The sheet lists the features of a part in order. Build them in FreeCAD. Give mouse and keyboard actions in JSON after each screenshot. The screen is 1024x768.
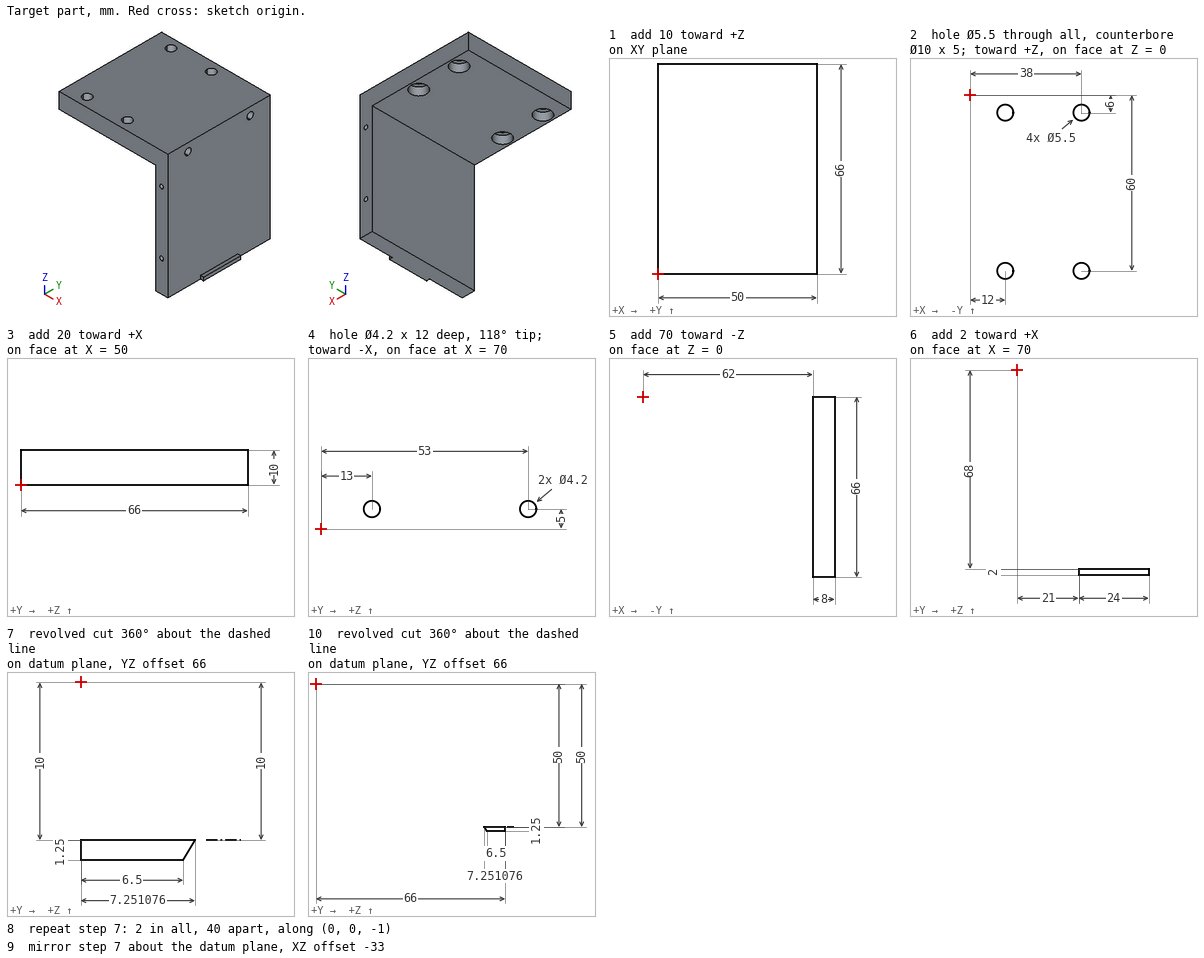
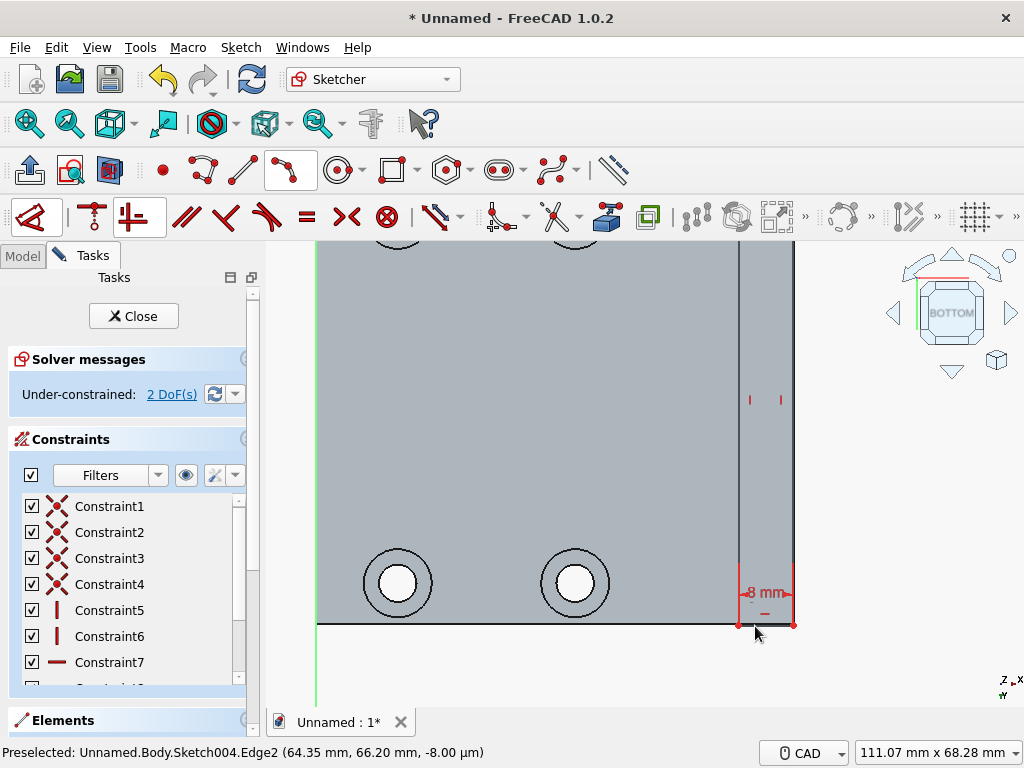
{"action": "left_click", "coordinate": [739, 309]}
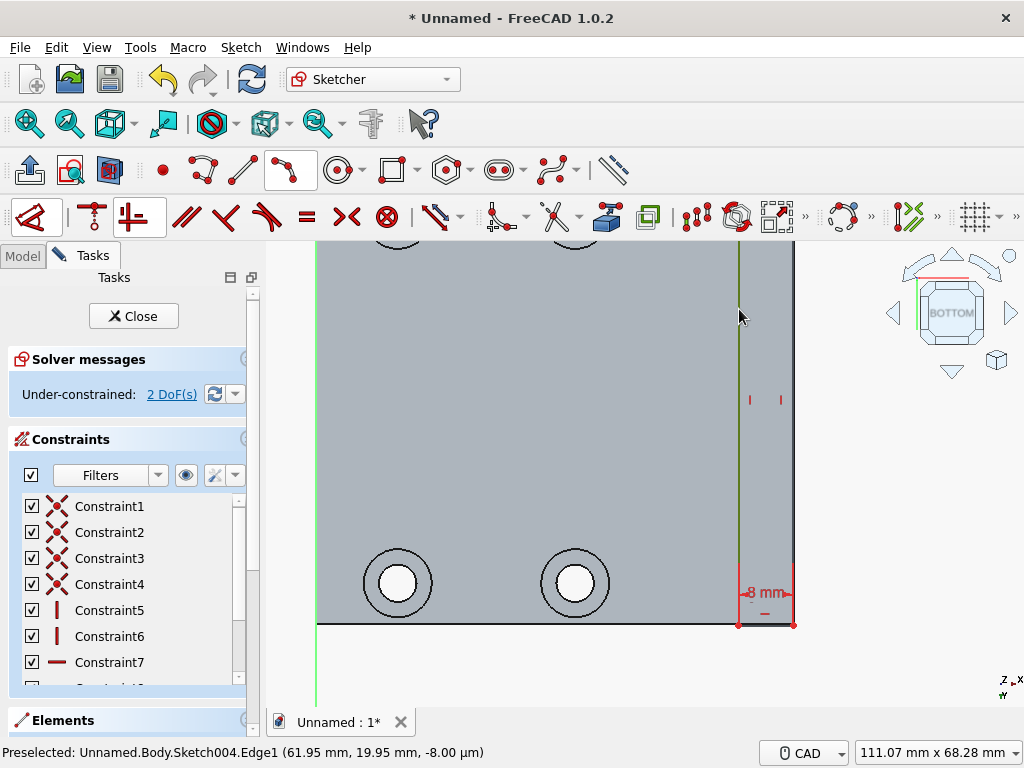
{"action": "key", "text": "i"}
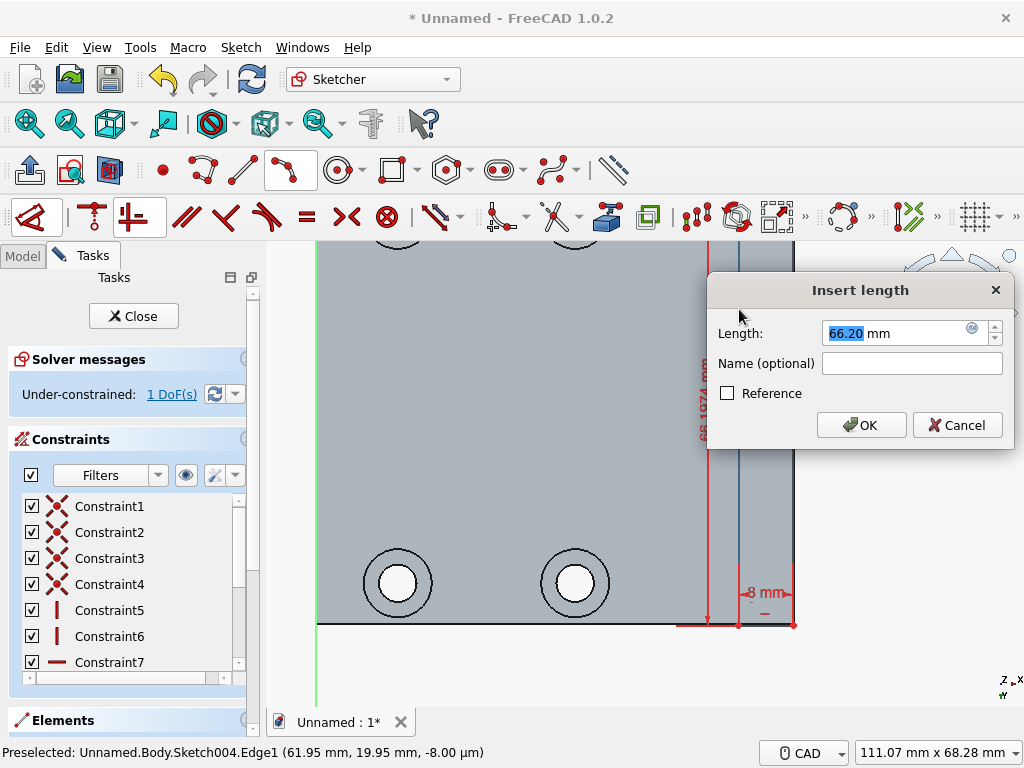
{"action": "type", "text": "66"}
{"action": "key", "text": "Return"}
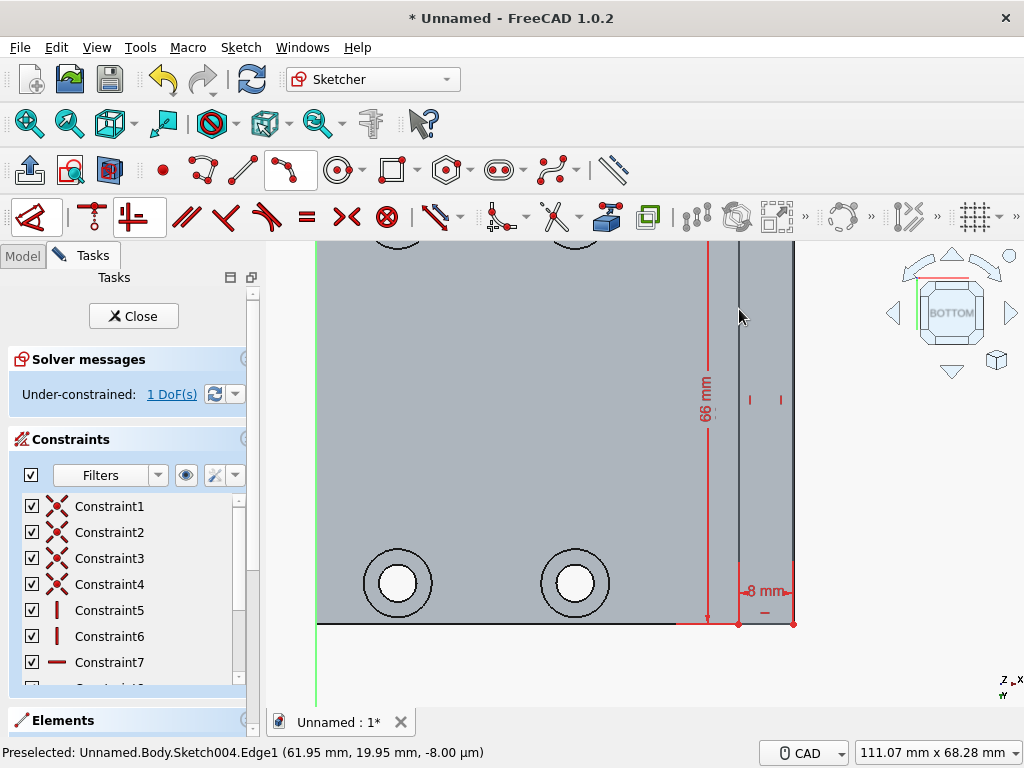
{"action": "scroll", "coordinate": [621, 626], "scroll_direction": "down", "scroll_amount": 2}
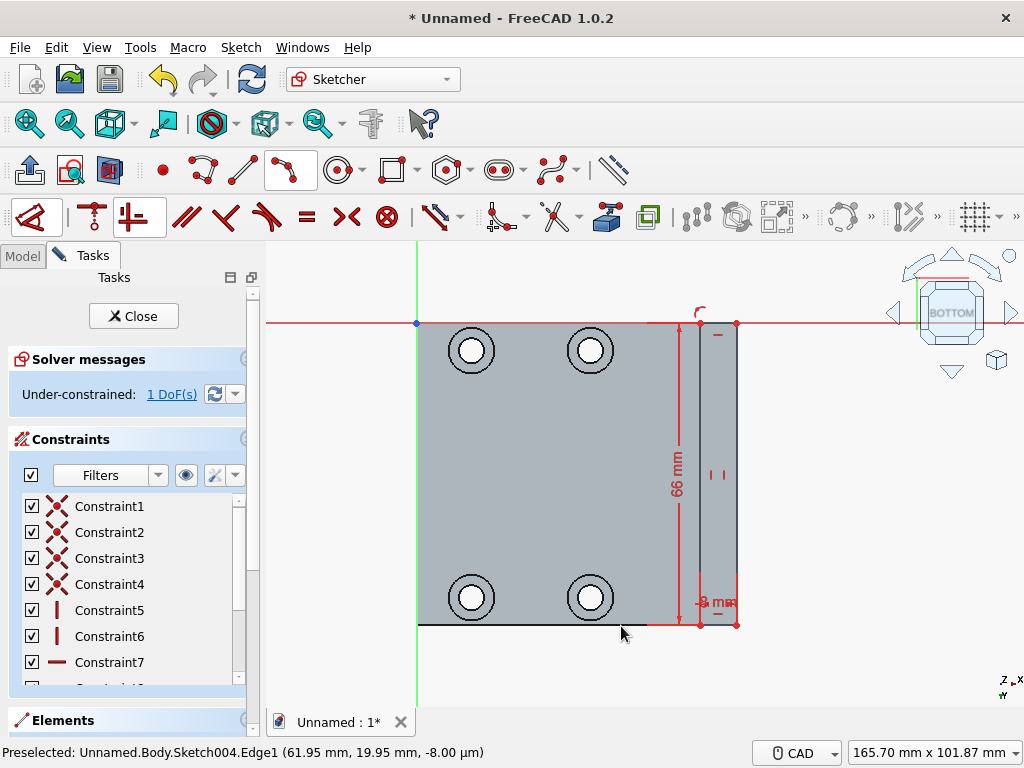
{"action": "left_click", "coordinate": [700, 323]}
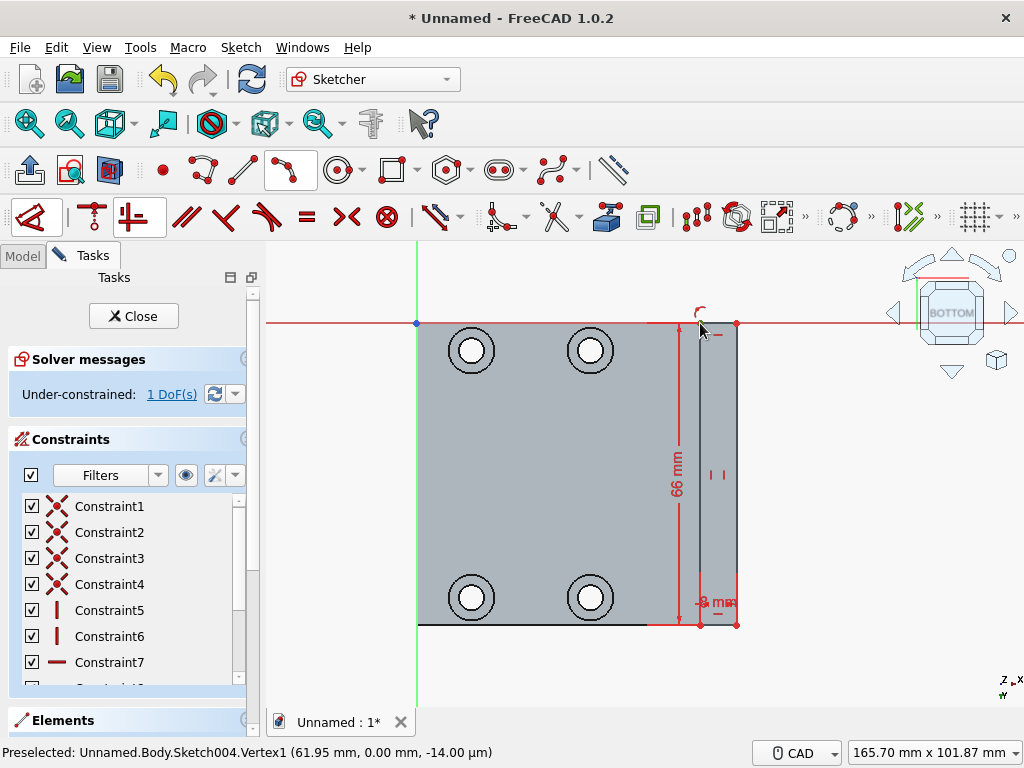
{"action": "key", "text": "l"}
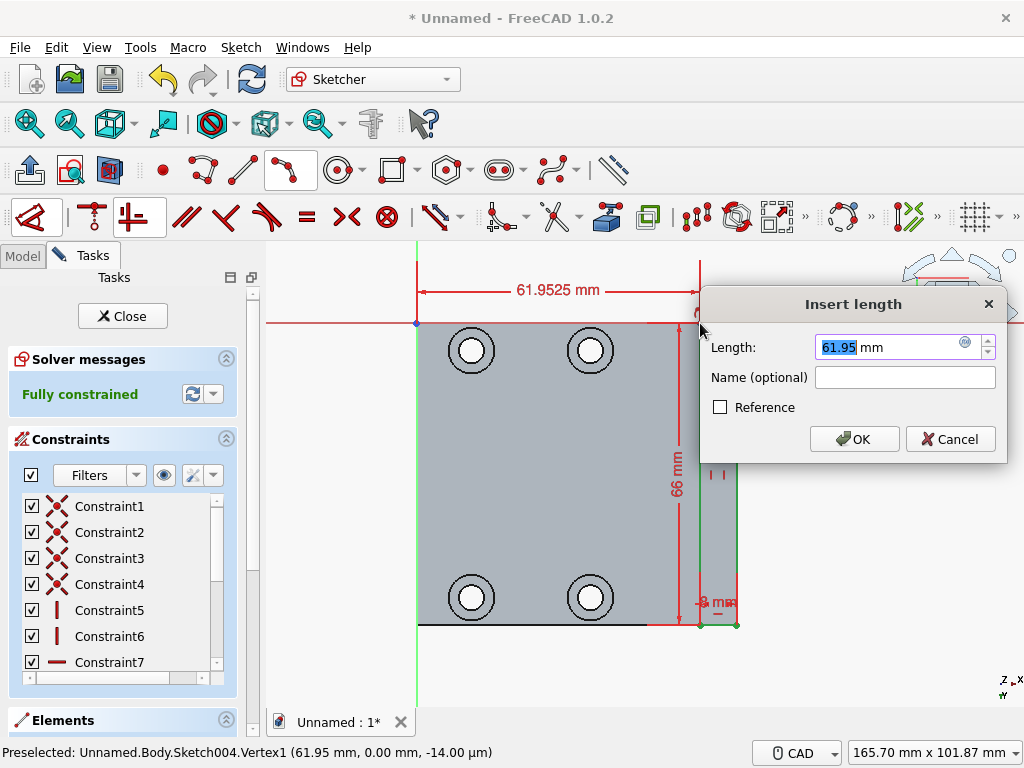
{"action": "type", "text": "62"}
{"action": "key", "text": "Return"}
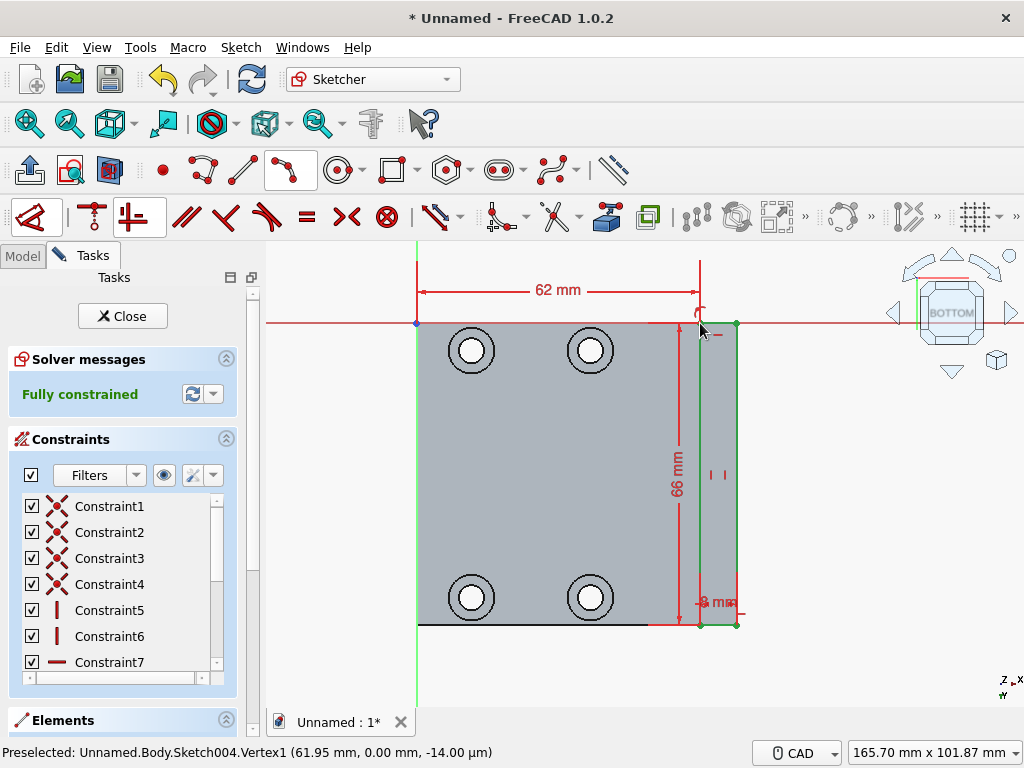
{"action": "left_click", "coordinate": [123, 316]}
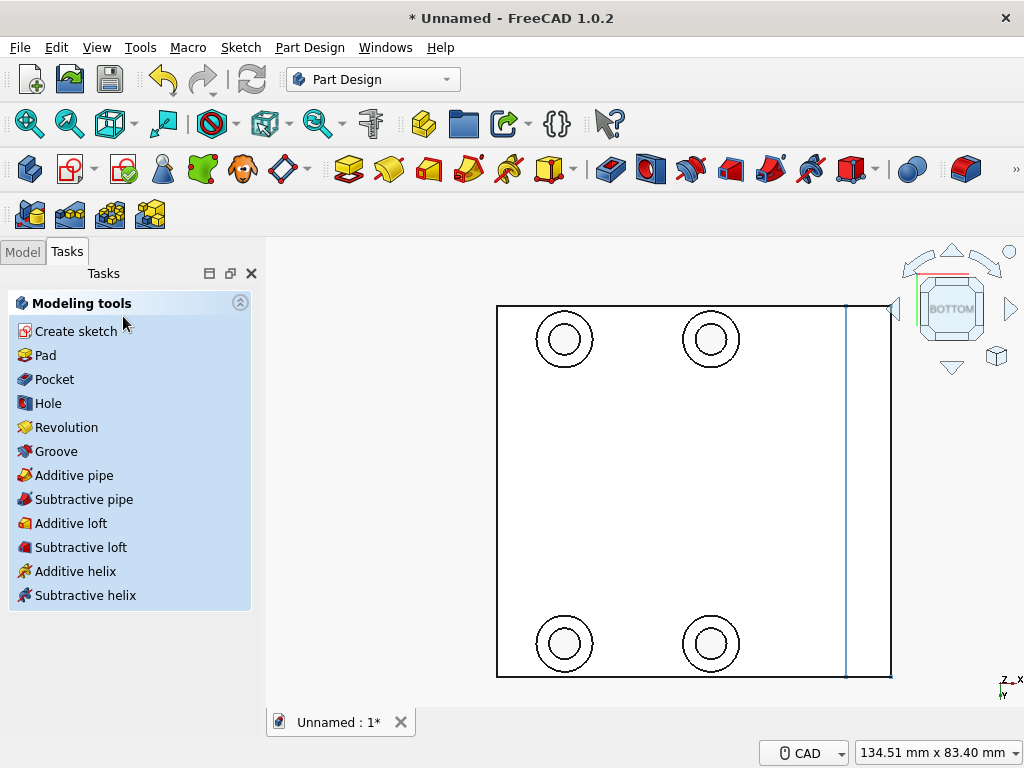
{"action": "left_click", "coordinate": [350, 170]}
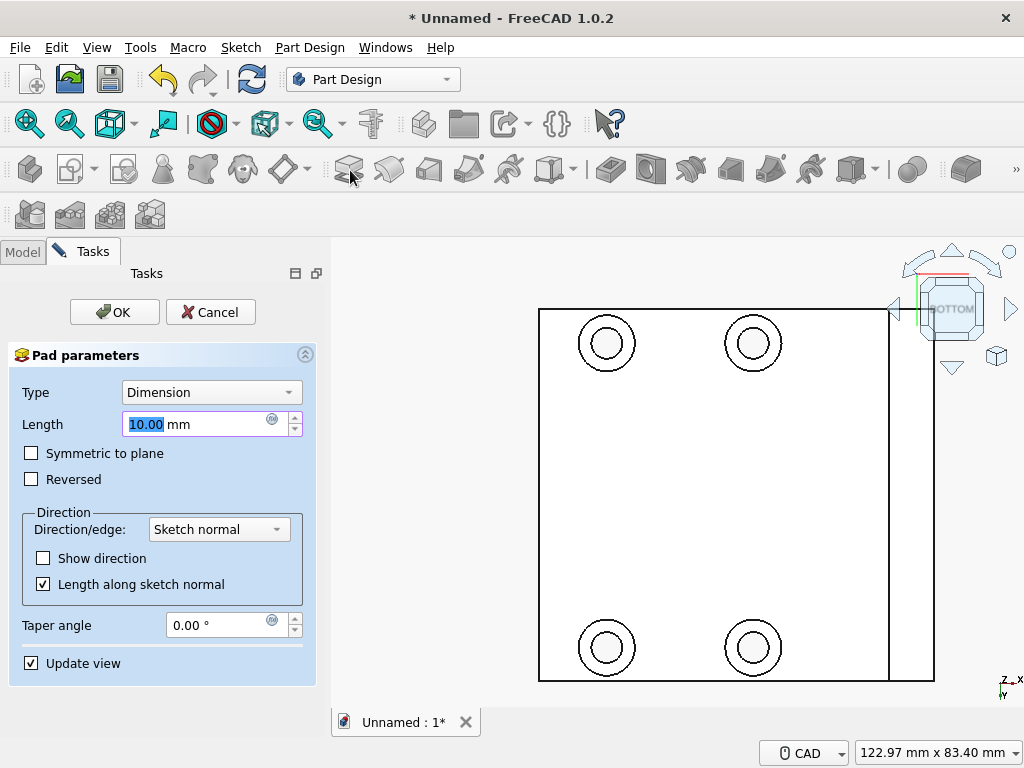
{"action": "type", "text": "70"}
{"action": "key", "text": "Tab"}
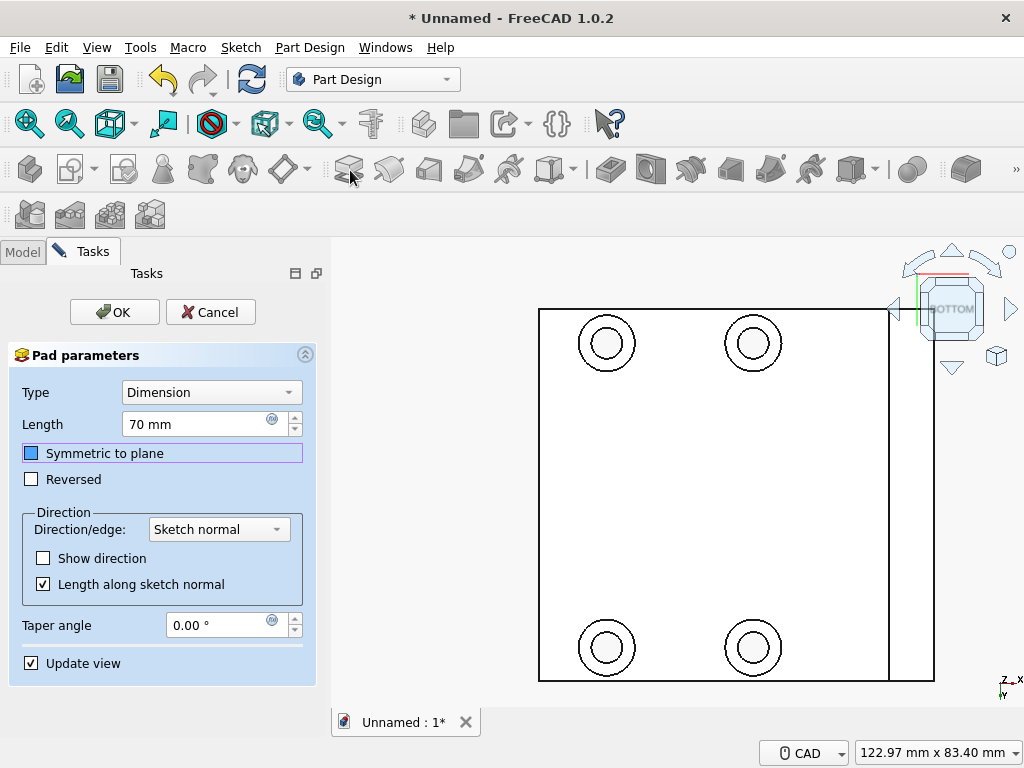
{"action": "left_click", "coordinate": [115, 312]}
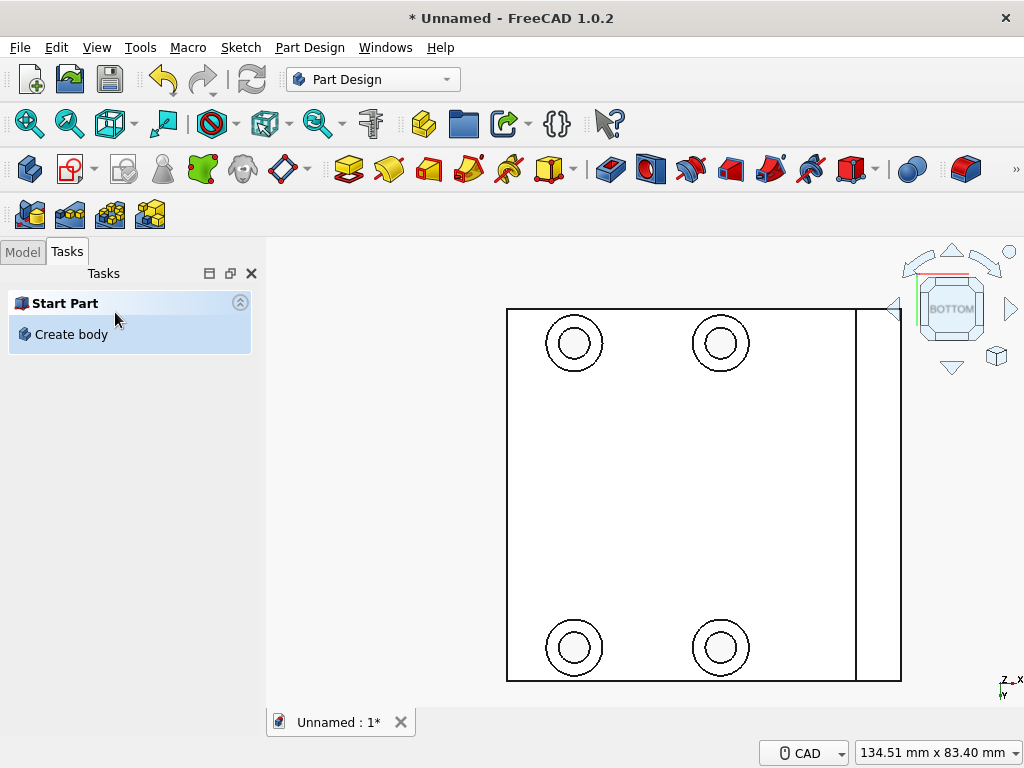
{"action": "key", "text": "0"}